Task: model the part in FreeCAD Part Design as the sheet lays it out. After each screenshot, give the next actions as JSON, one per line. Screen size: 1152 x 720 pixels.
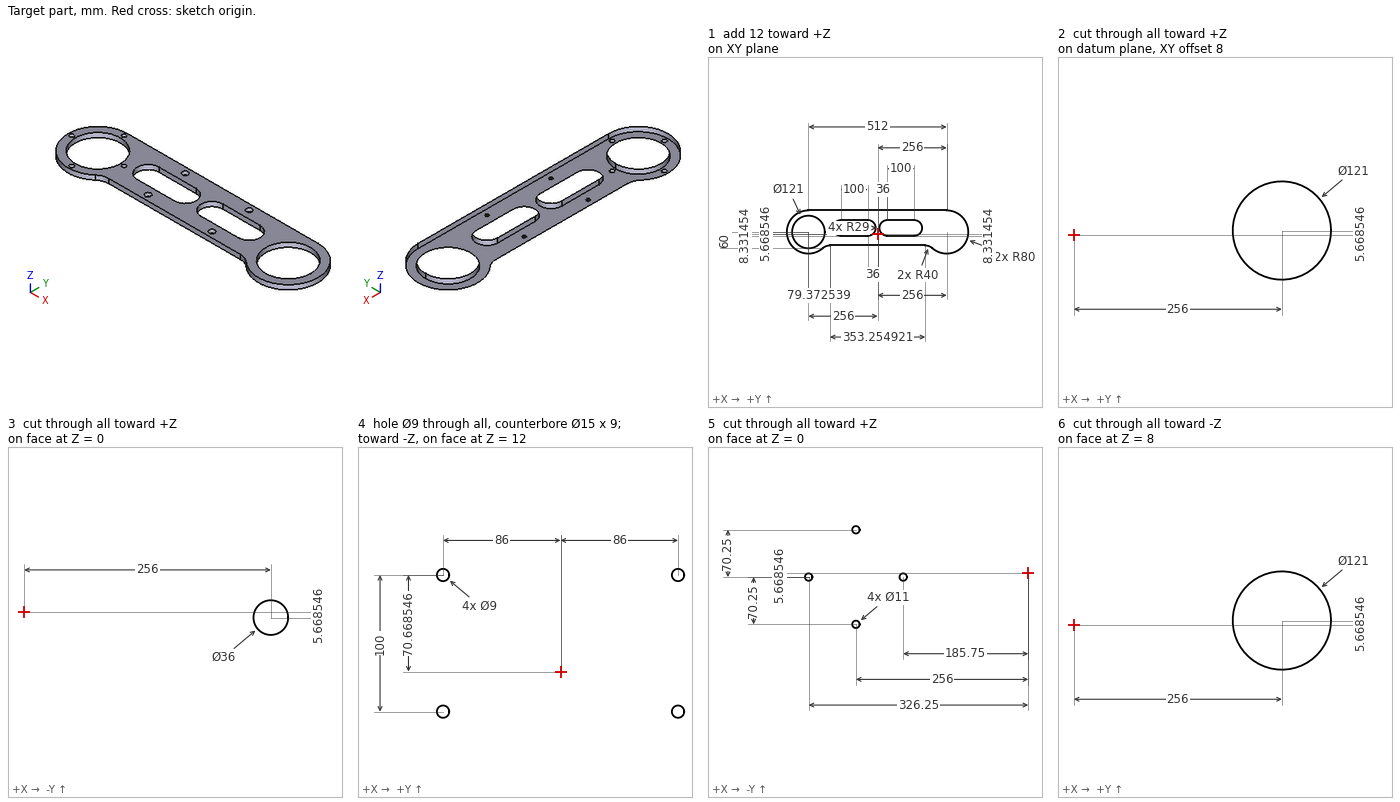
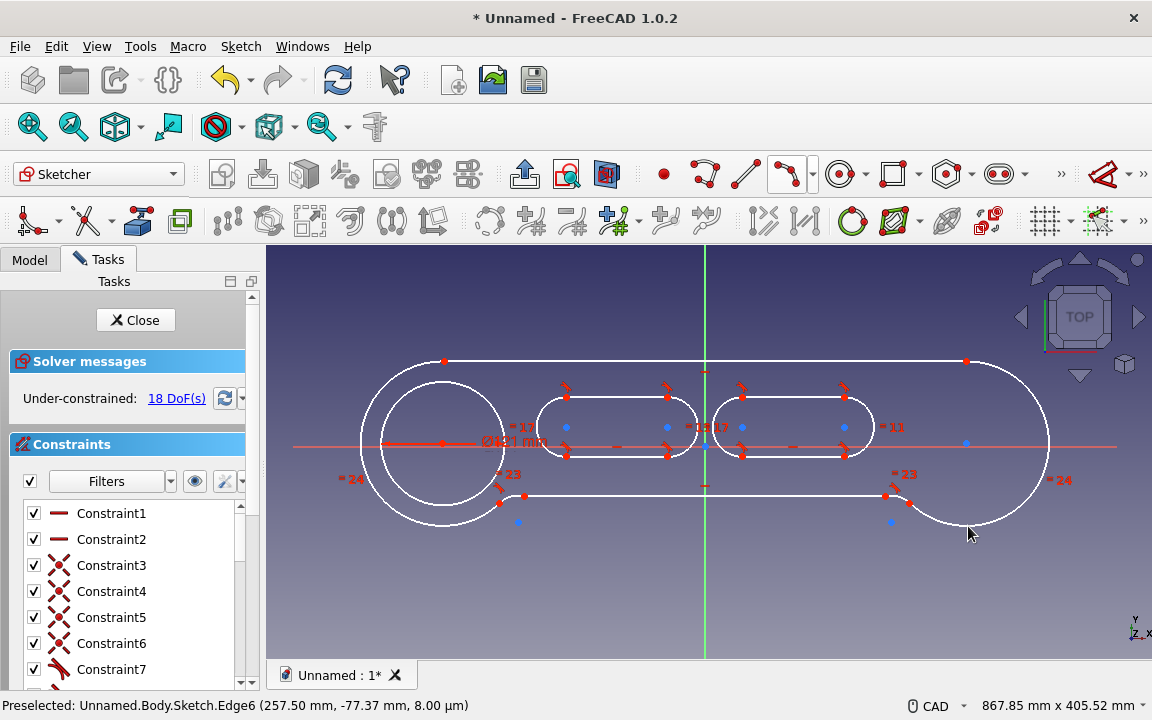
{"action": "left_click", "coordinate": [718, 410]}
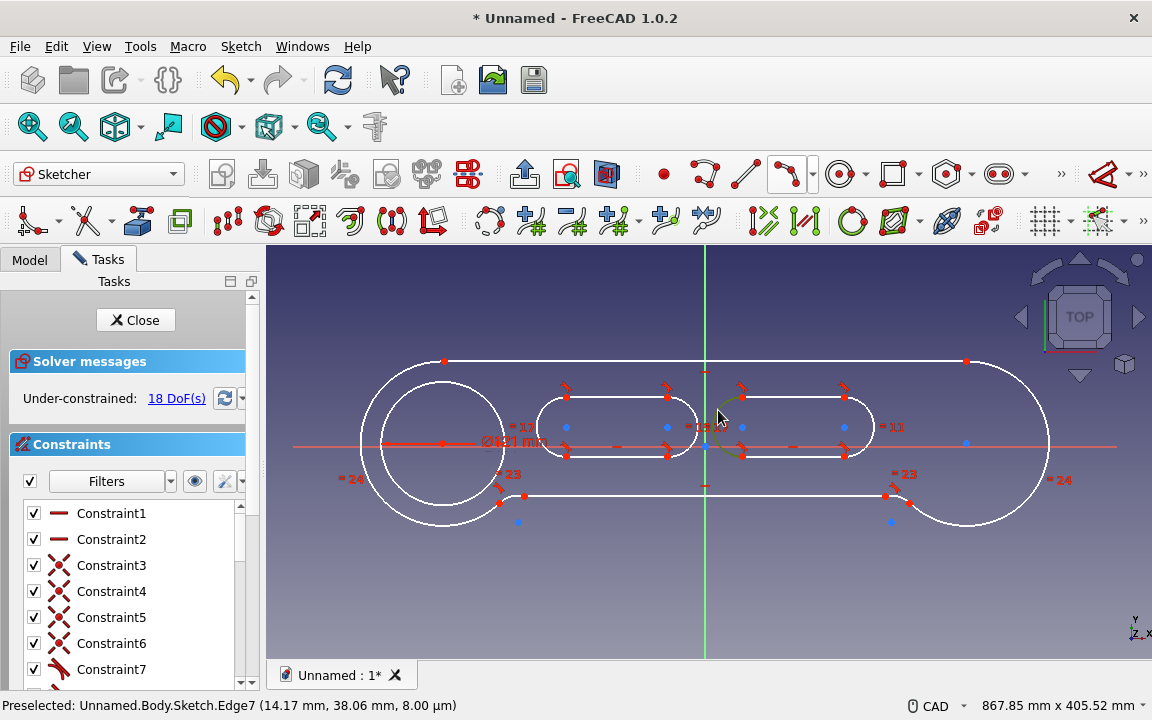
{"action": "left_click", "coordinate": [542, 410]}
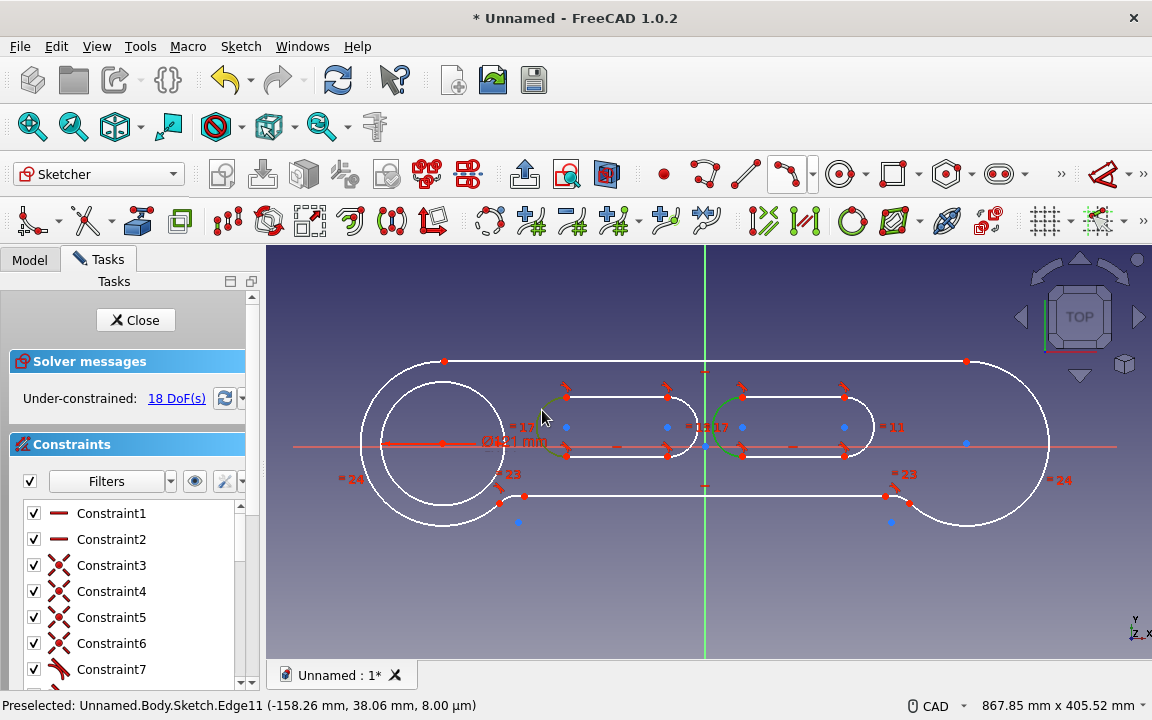
{"action": "key", "text": "e"}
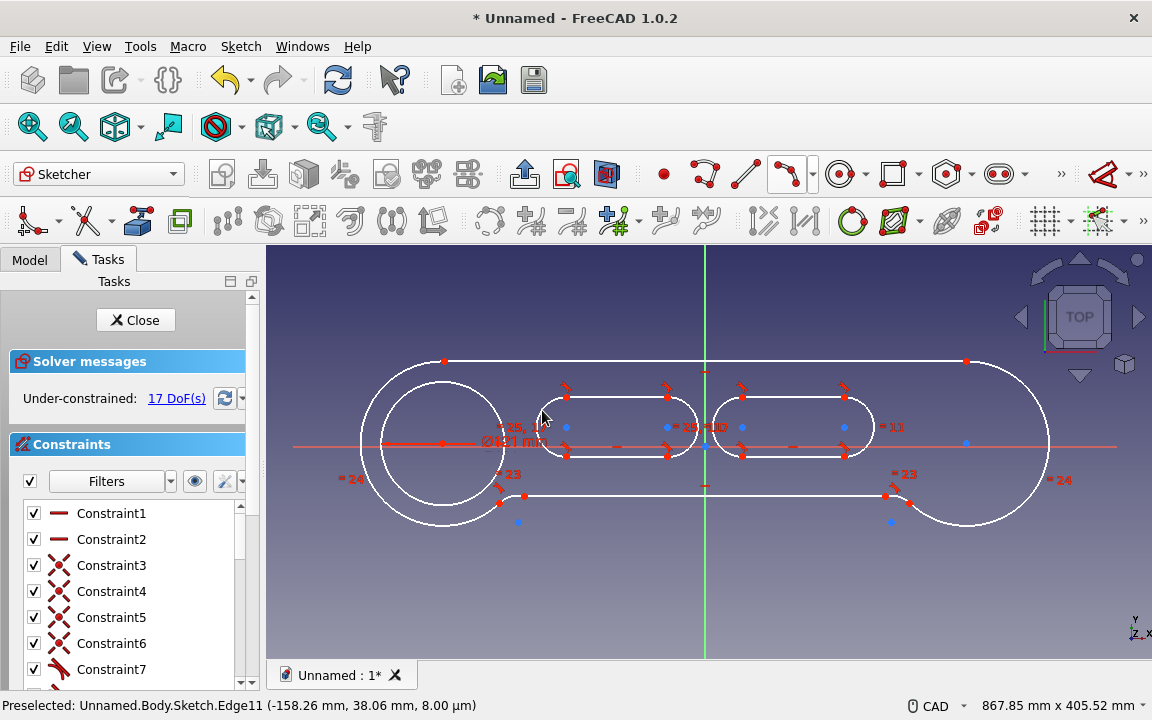
{"action": "left_click", "coordinate": [1102, 174]}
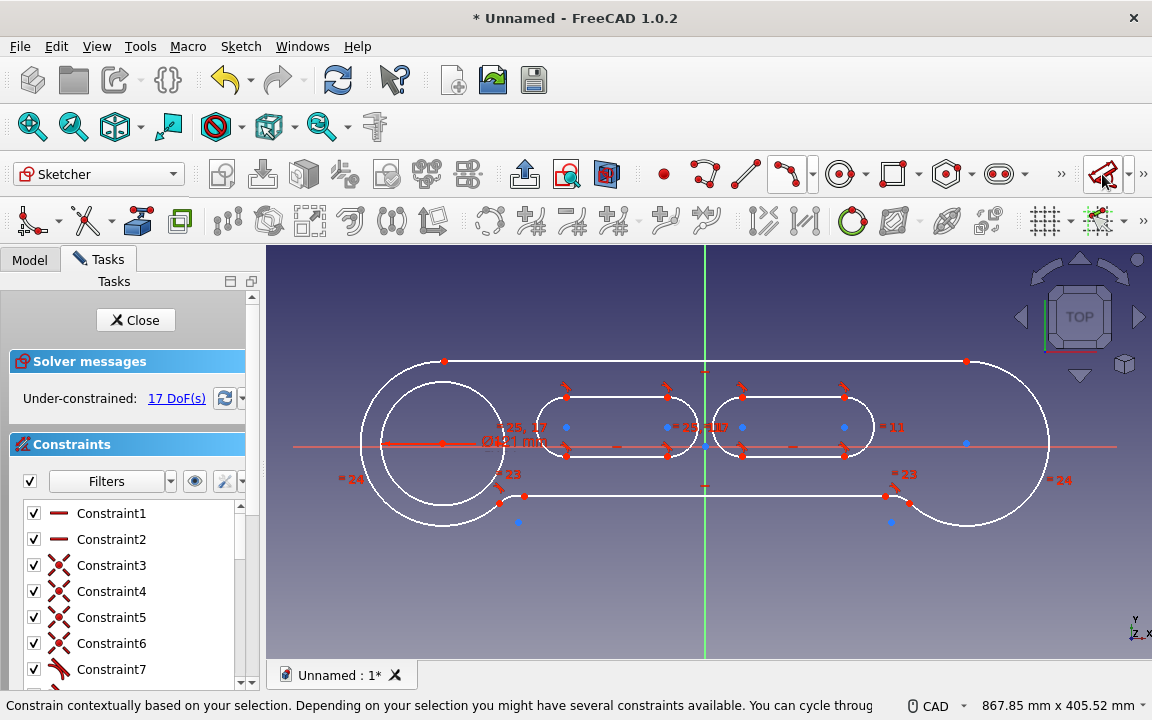
{"action": "left_click", "coordinate": [367, 411]}
{"action": "left_click", "coordinate": [338, 398]}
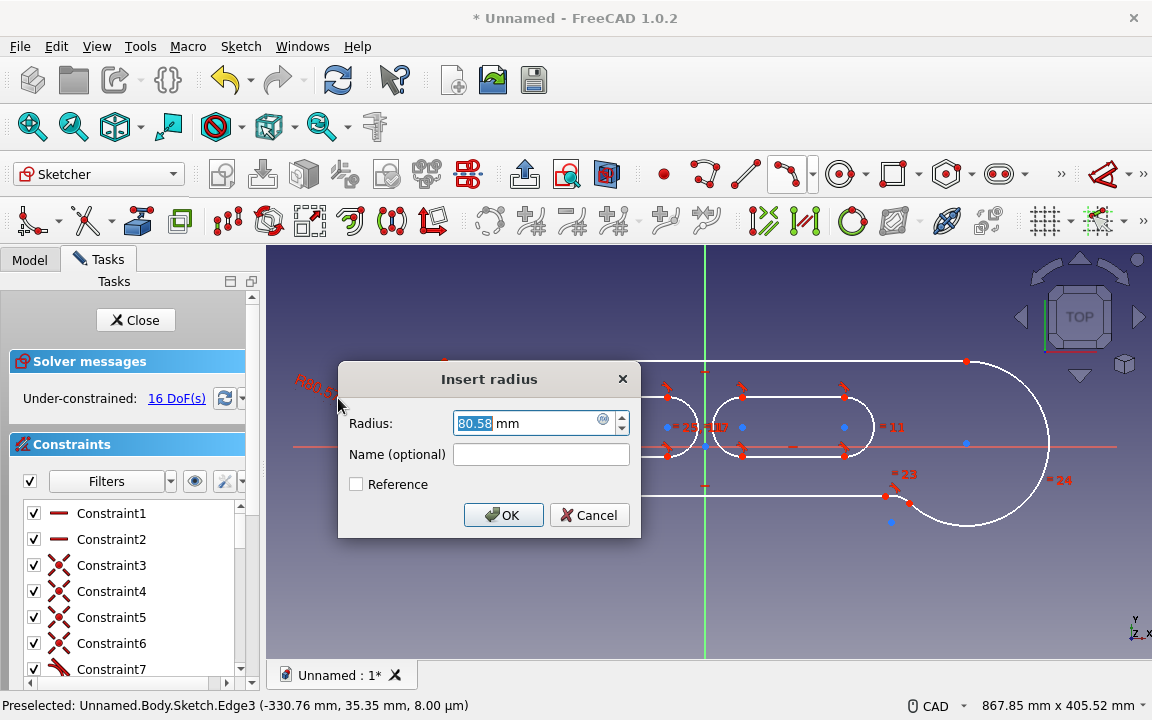
{"action": "type", "text": "80"}
{"action": "key", "text": "Return"}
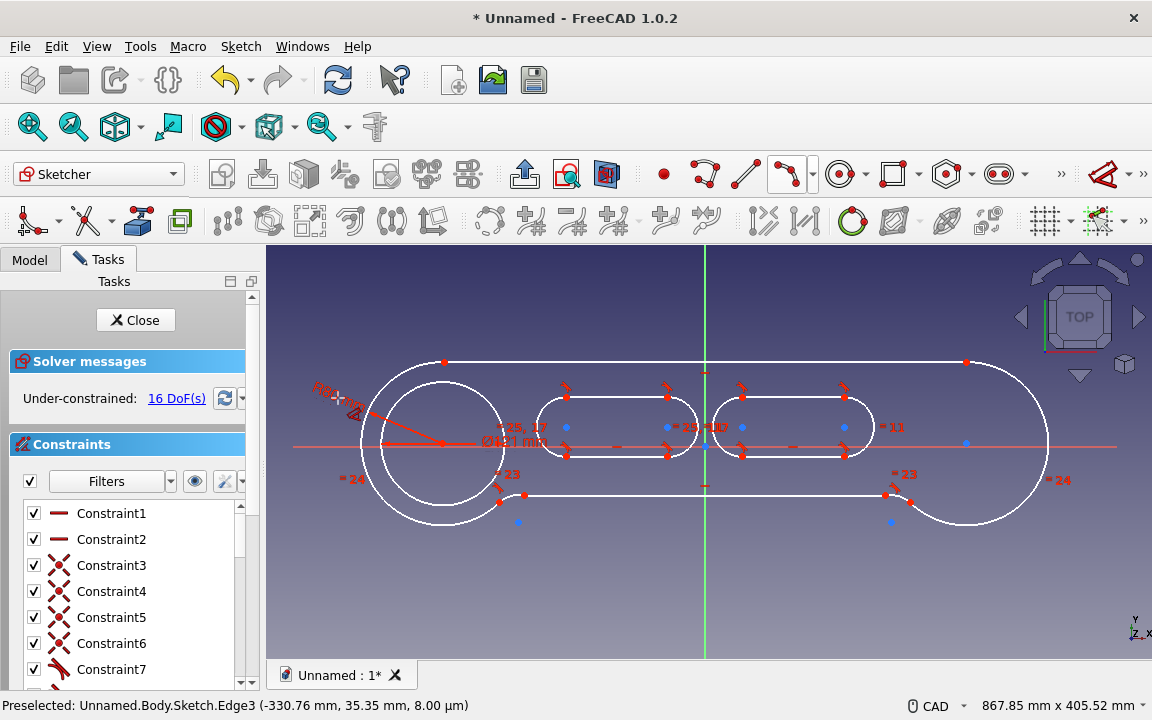
{"action": "left_click", "coordinate": [511, 496]}
{"action": "left_click", "coordinate": [532, 464]}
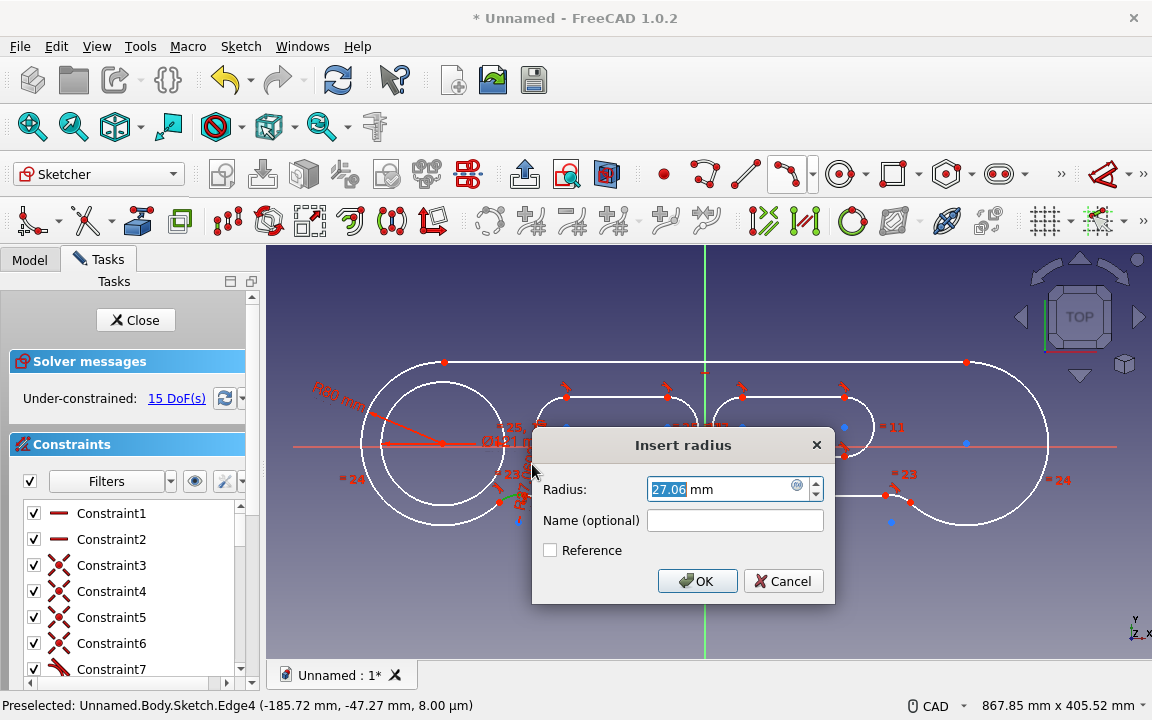
{"action": "type", "text": "40"}
{"action": "key", "text": "Return"}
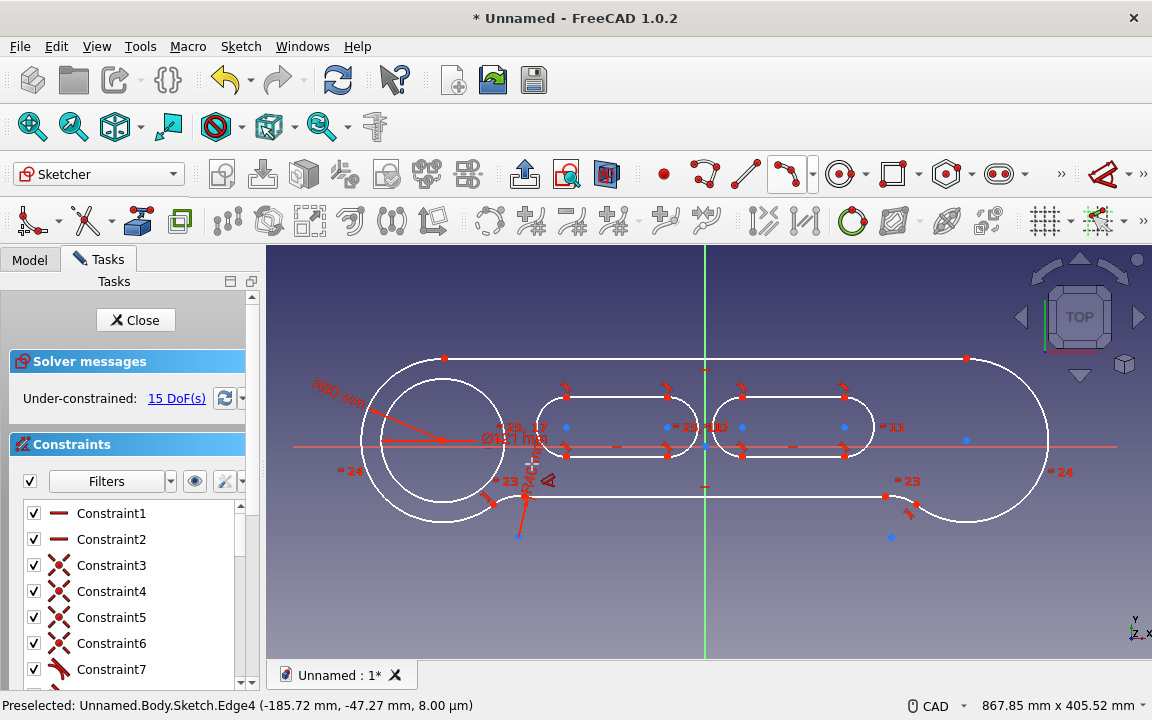
{"action": "scroll", "coordinate": [718, 410], "scroll_direction": "up", "scroll_amount": 2}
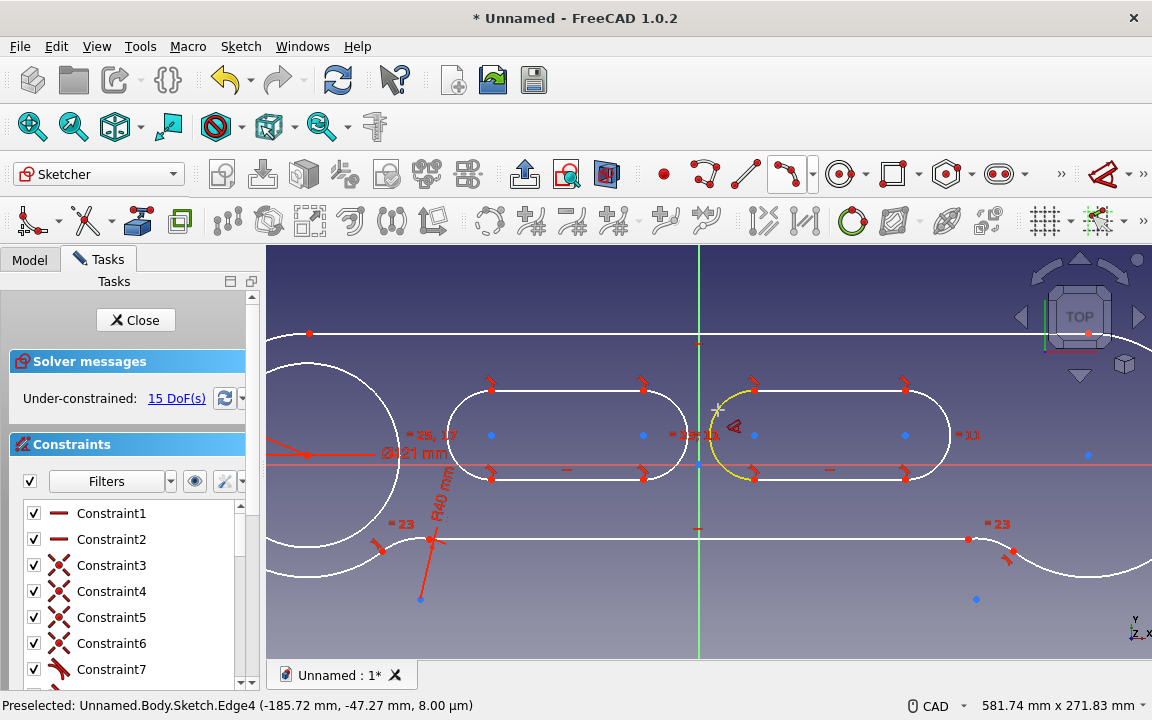
{"action": "left_click", "coordinate": [718, 409]}
{"action": "left_click", "coordinate": [721, 366]}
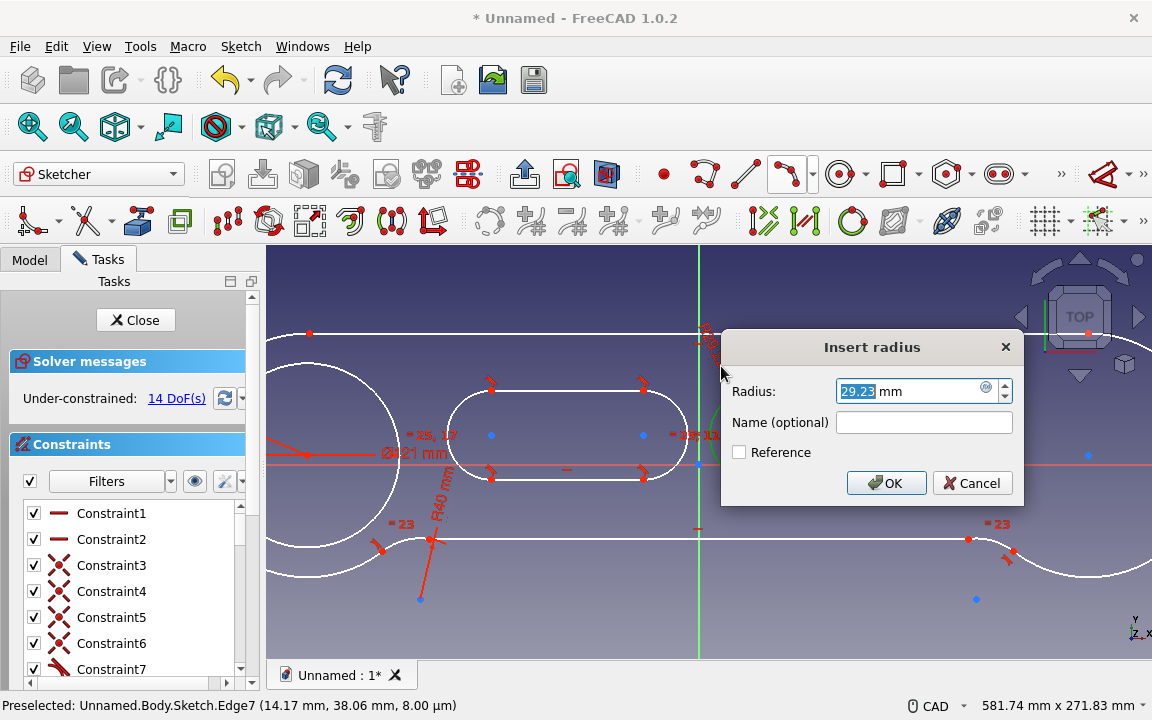
{"action": "type", "text": "29"}
{"action": "key", "text": "Return"}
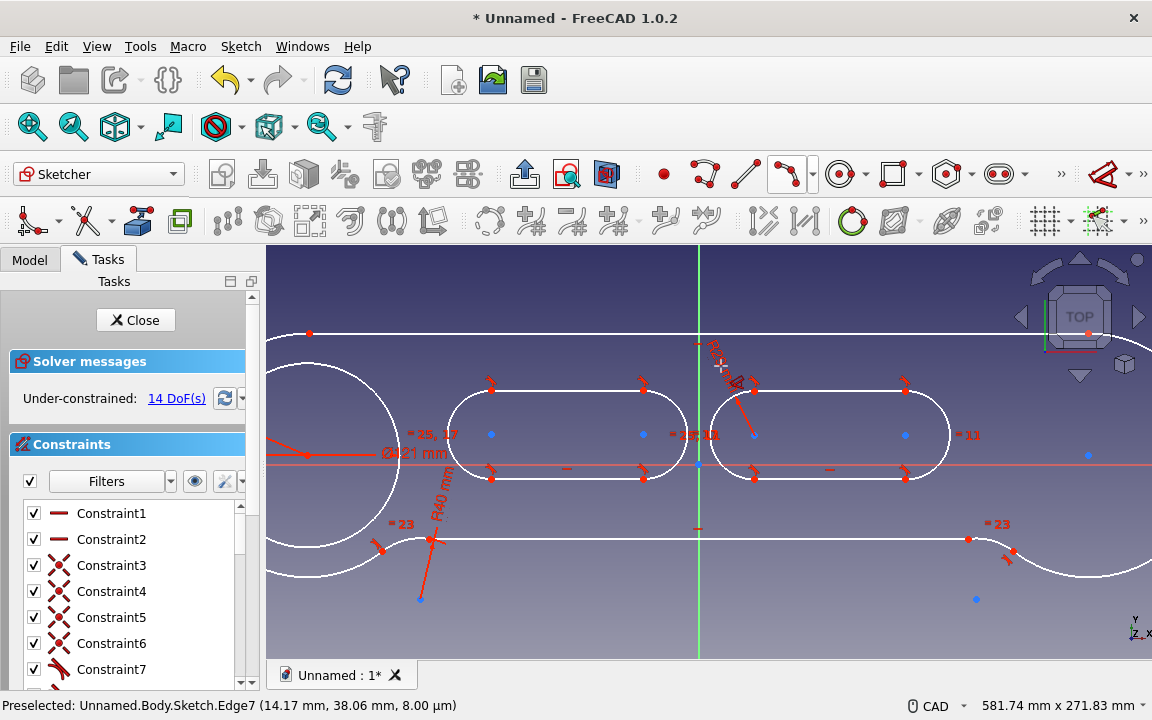
{"action": "left_click", "coordinate": [855, 334]}
{"action": "left_click", "coordinate": [648, 300]}